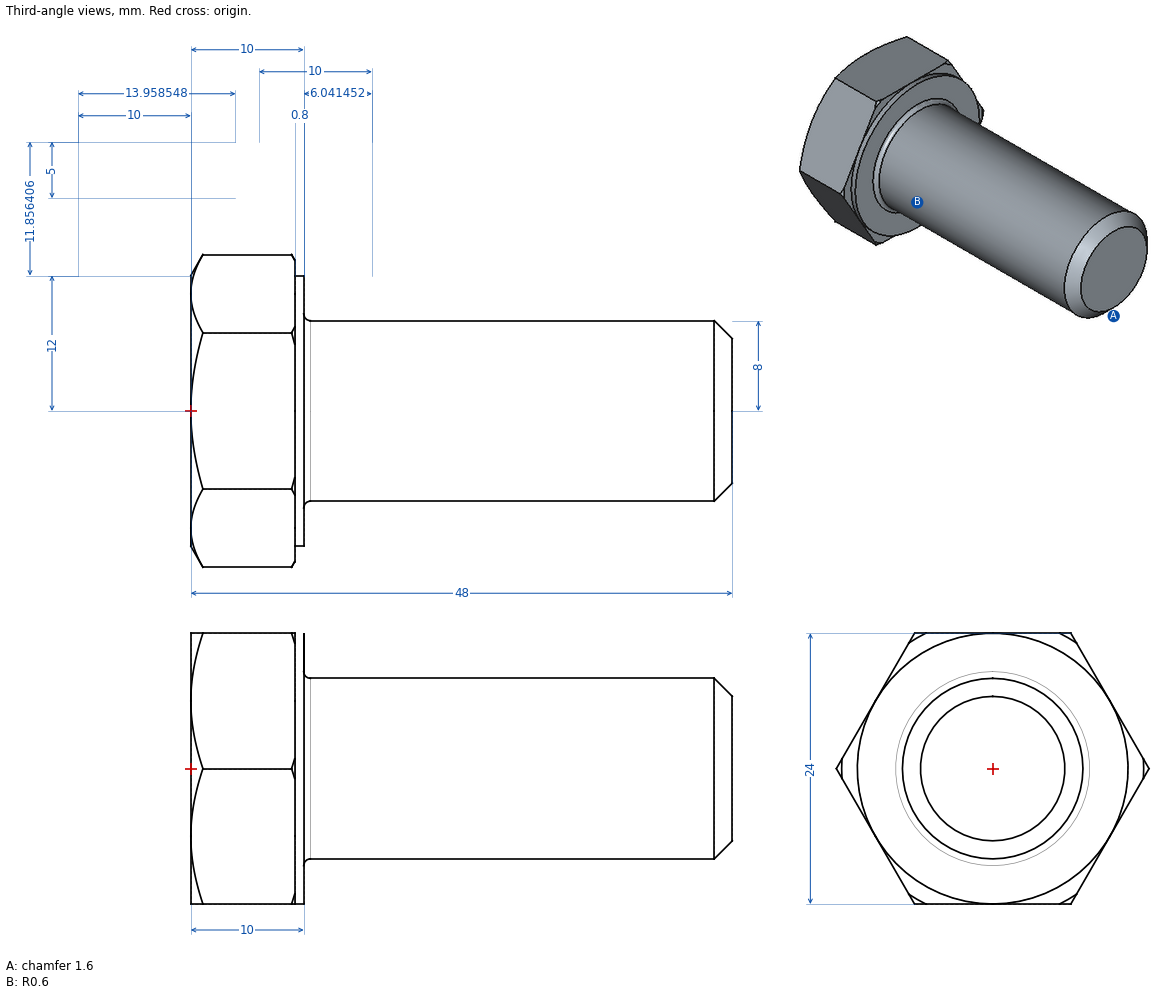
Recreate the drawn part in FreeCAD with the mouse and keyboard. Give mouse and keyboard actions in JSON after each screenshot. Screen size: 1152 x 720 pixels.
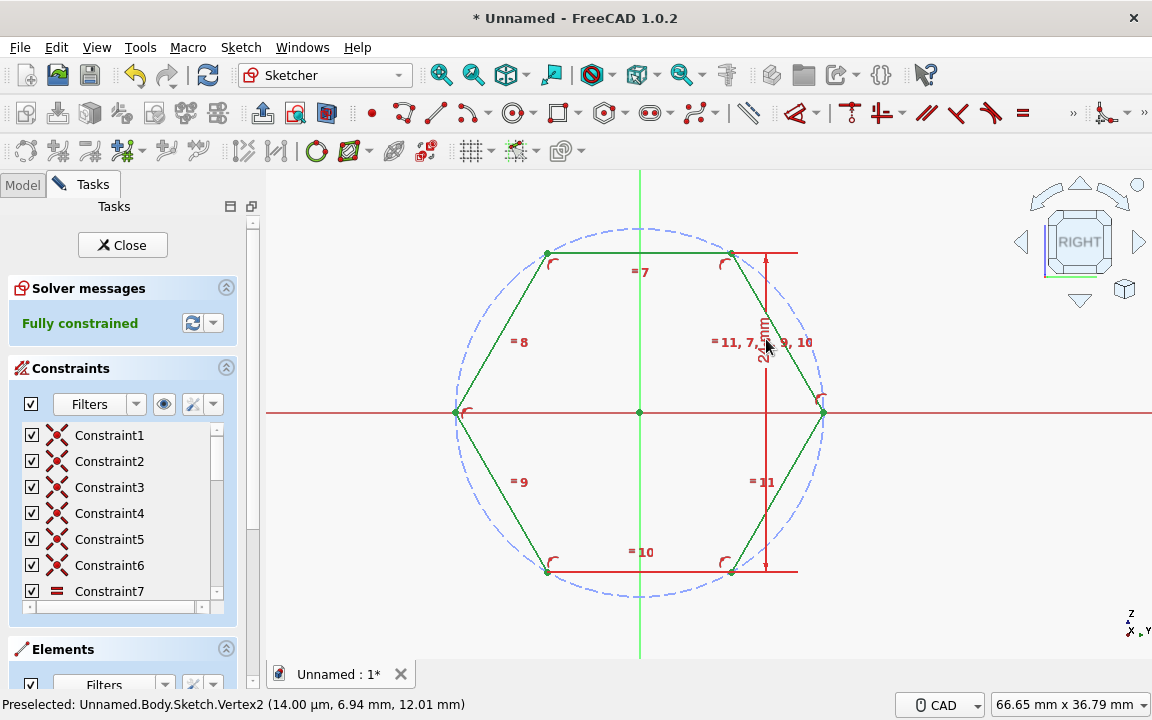
{"action": "left_click", "coordinate": [123, 245]}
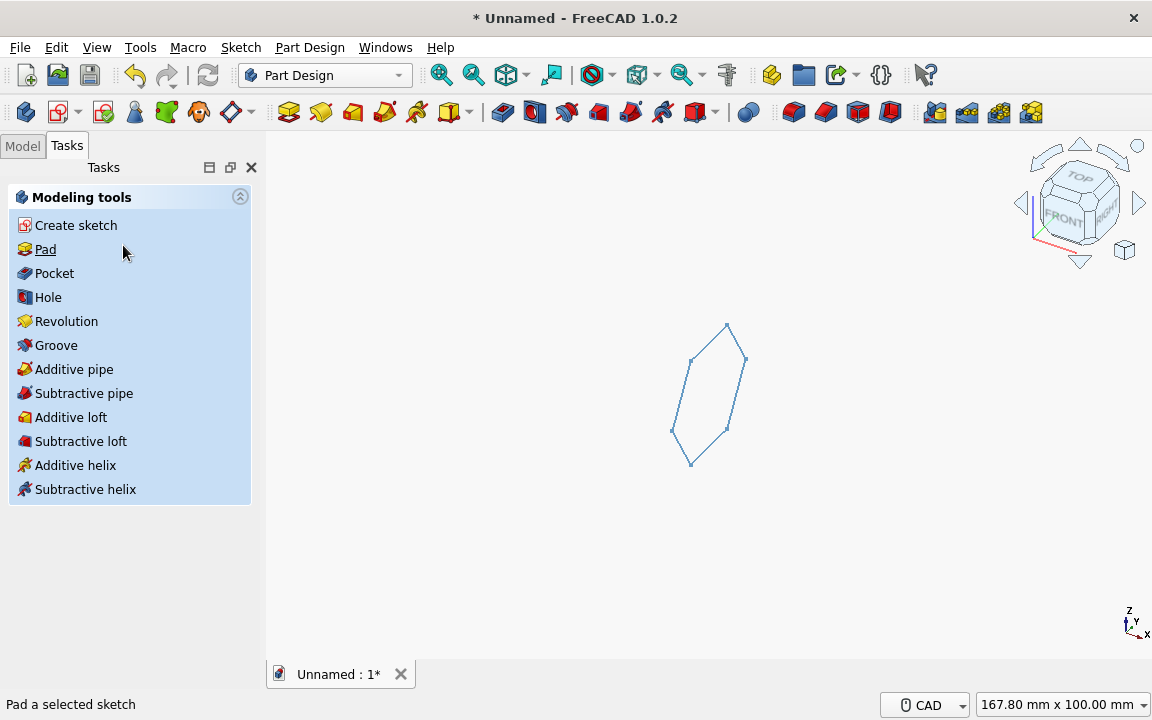
{"action": "left_click", "coordinate": [290, 112]}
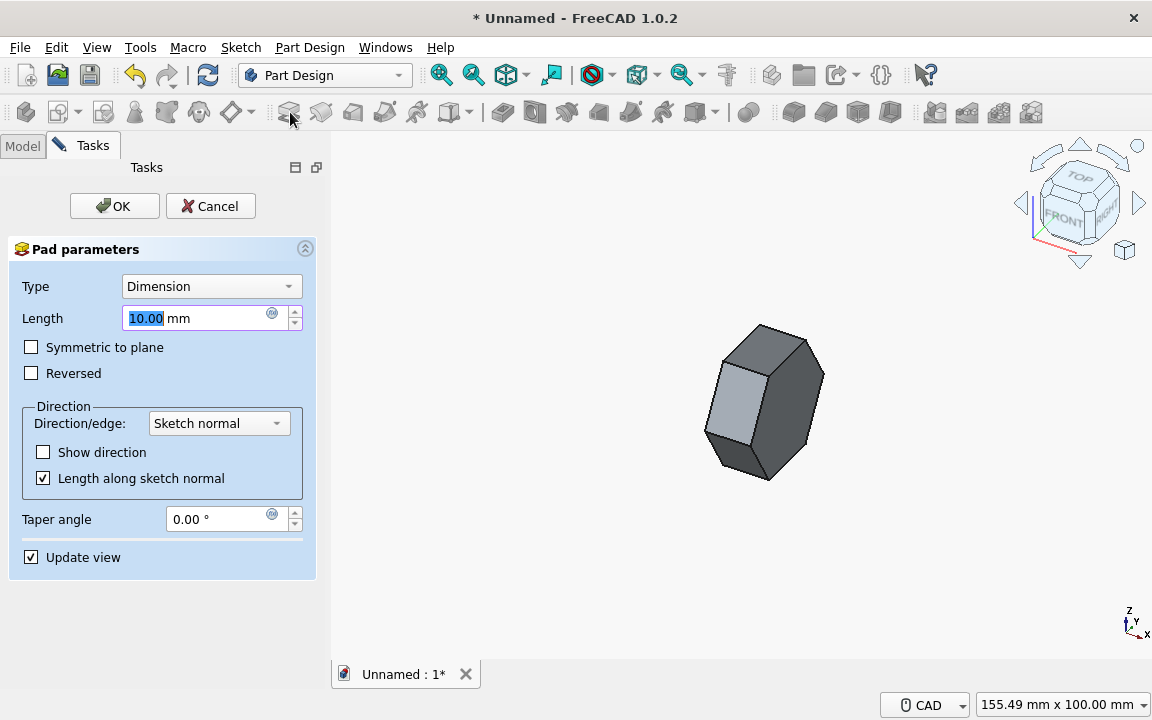
{"action": "type", "text": "10"}
{"action": "key", "text": "Tab"}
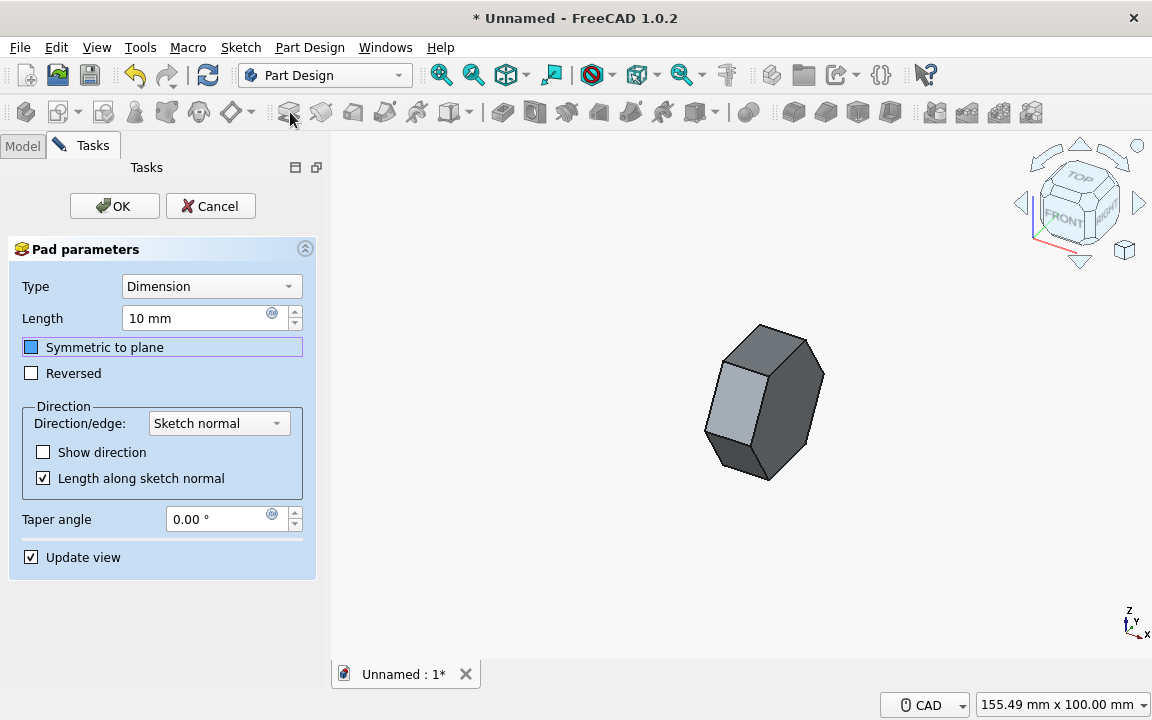
{"action": "left_click", "coordinate": [115, 206]}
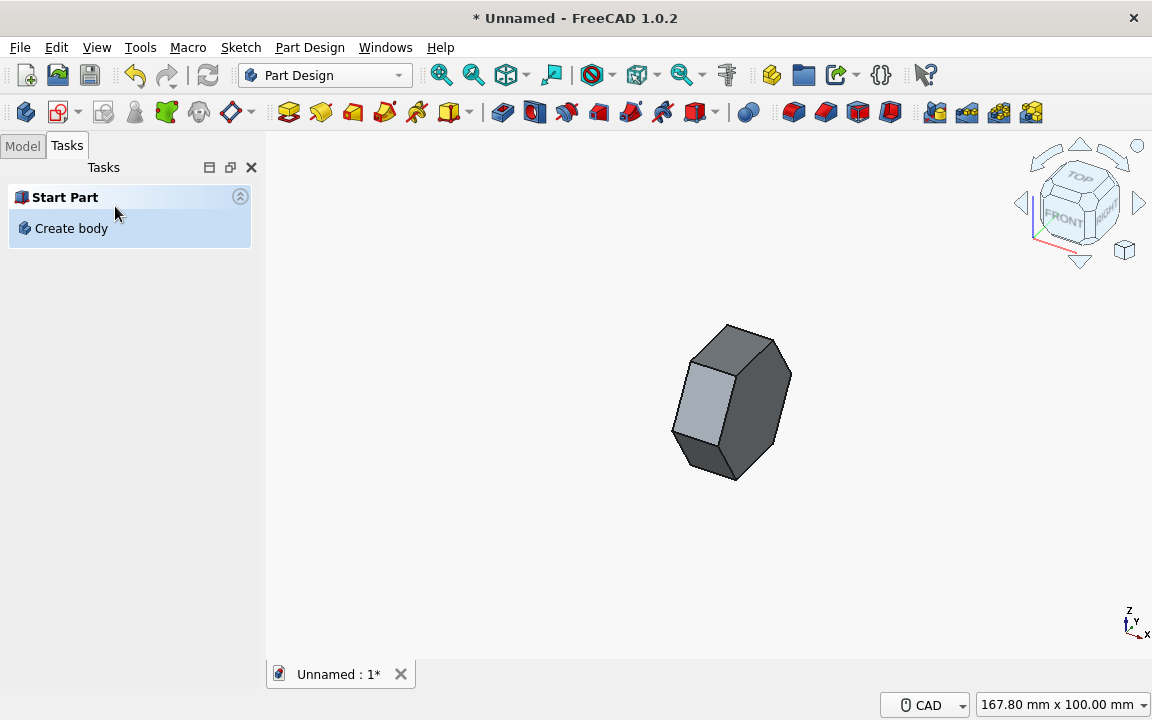
{"action": "left_click", "coordinate": [442, 76]}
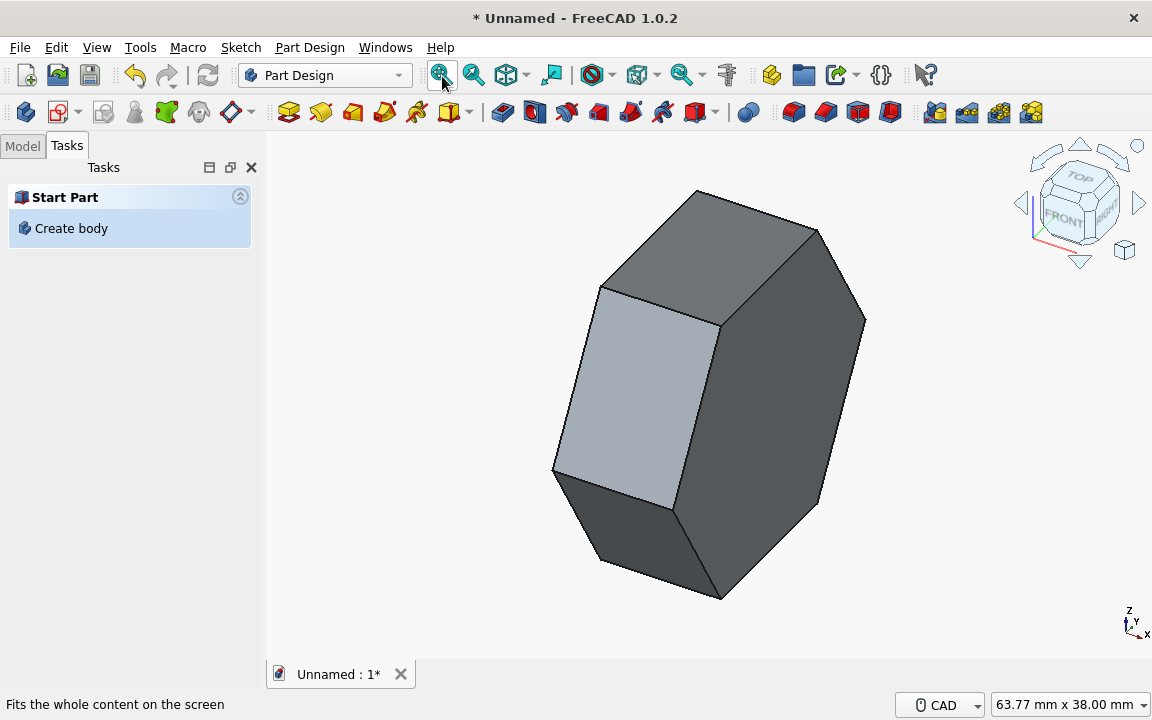
{"action": "left_click", "coordinate": [58, 112]}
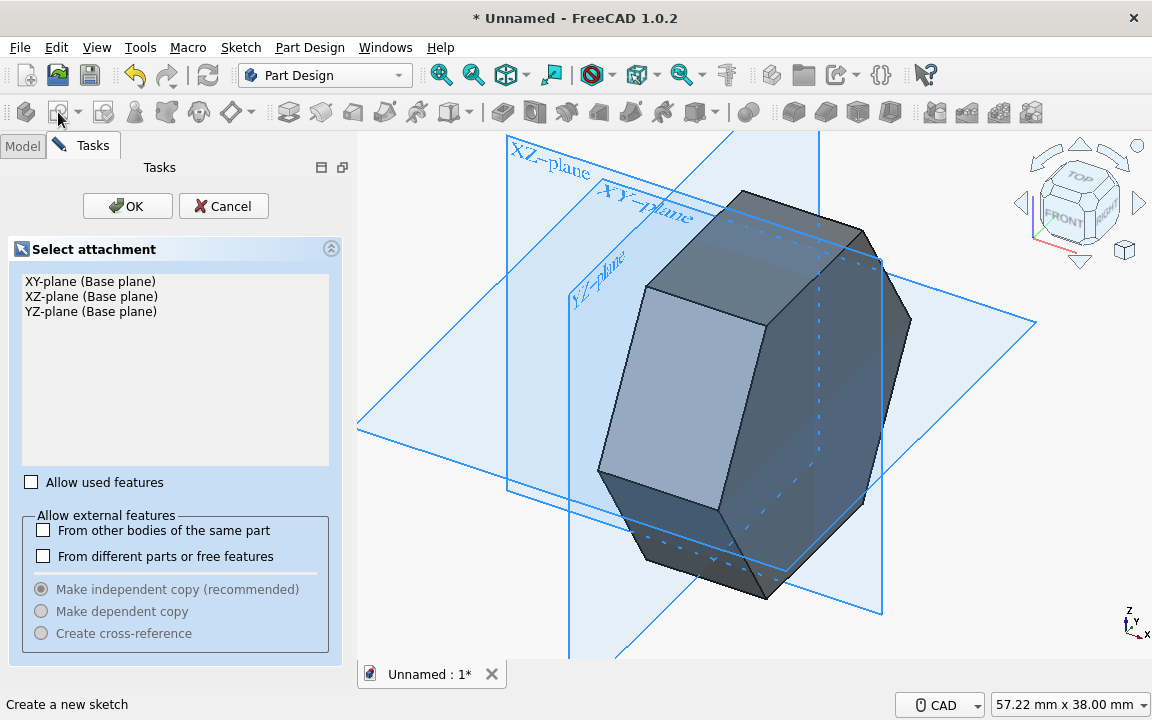
{"action": "left_click", "coordinate": [82, 282]}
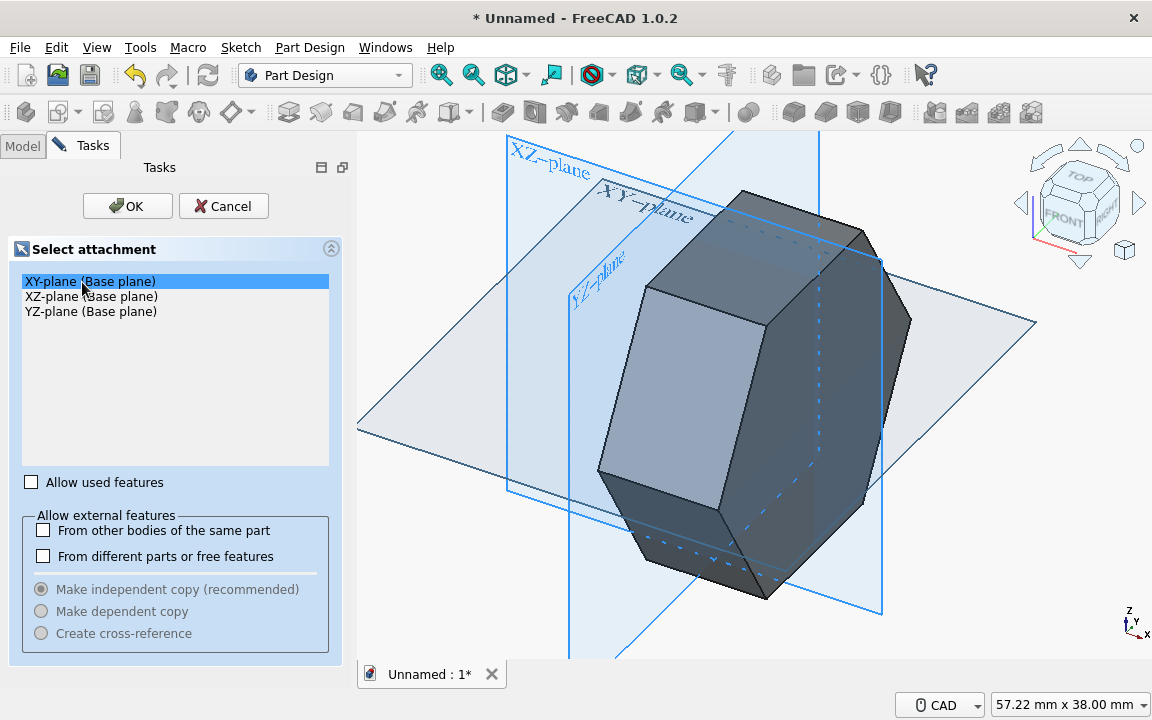
{"action": "left_click", "coordinate": [128, 206]}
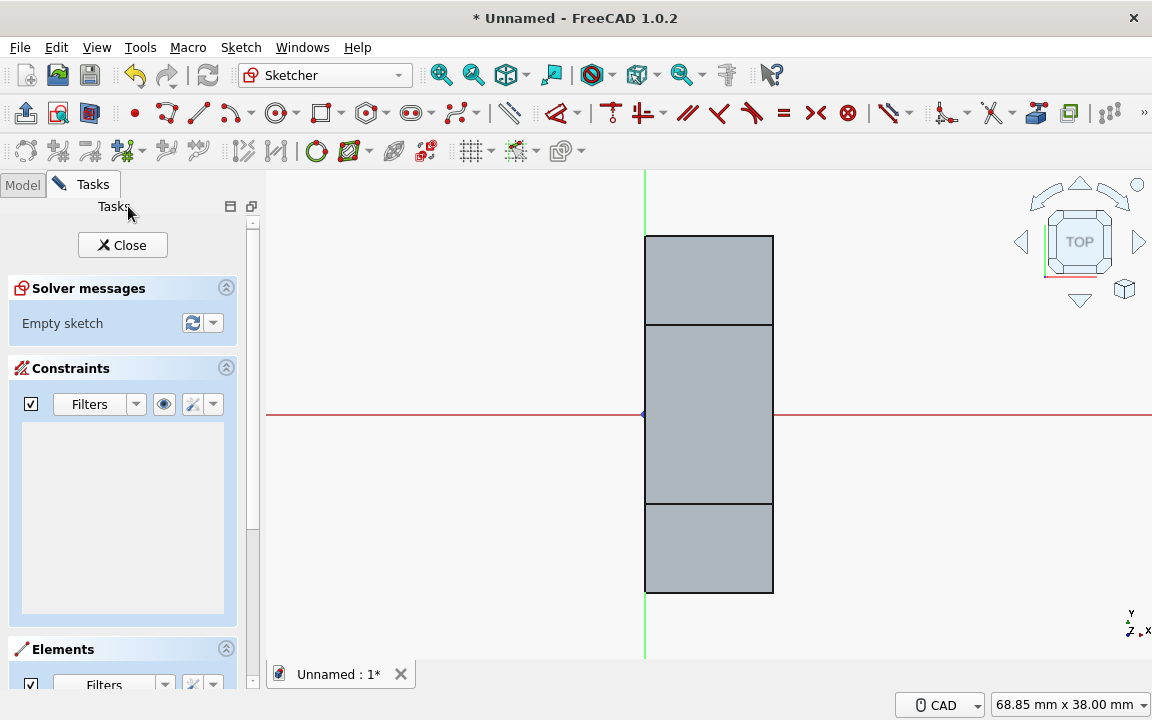
{"action": "left_click", "coordinate": [90, 114]}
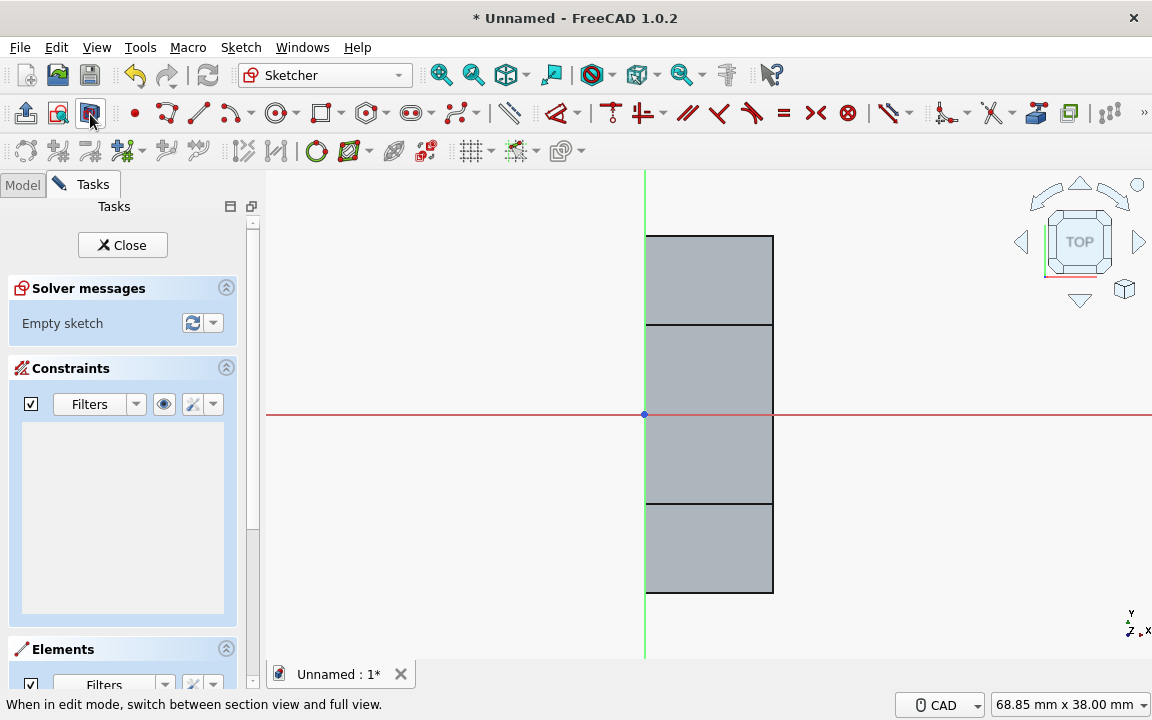
{"action": "scroll", "coordinate": [294, 519], "scroll_direction": "down", "scroll_amount": 2}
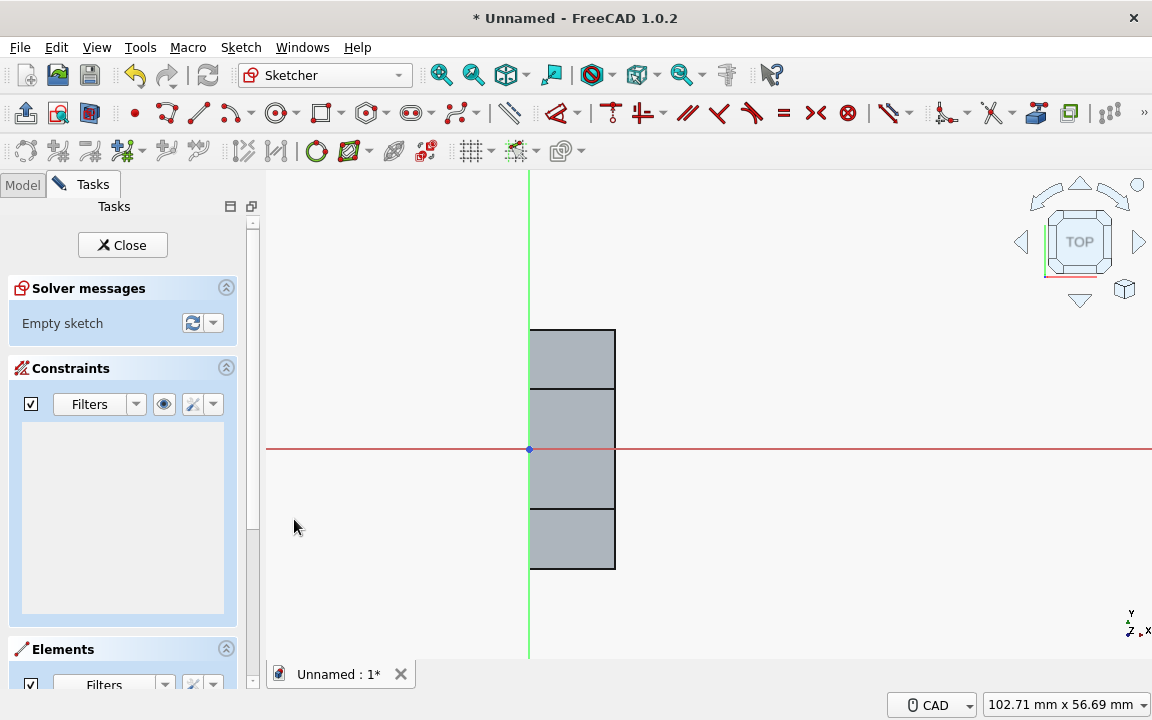
{"action": "left_click", "coordinate": [322, 114]}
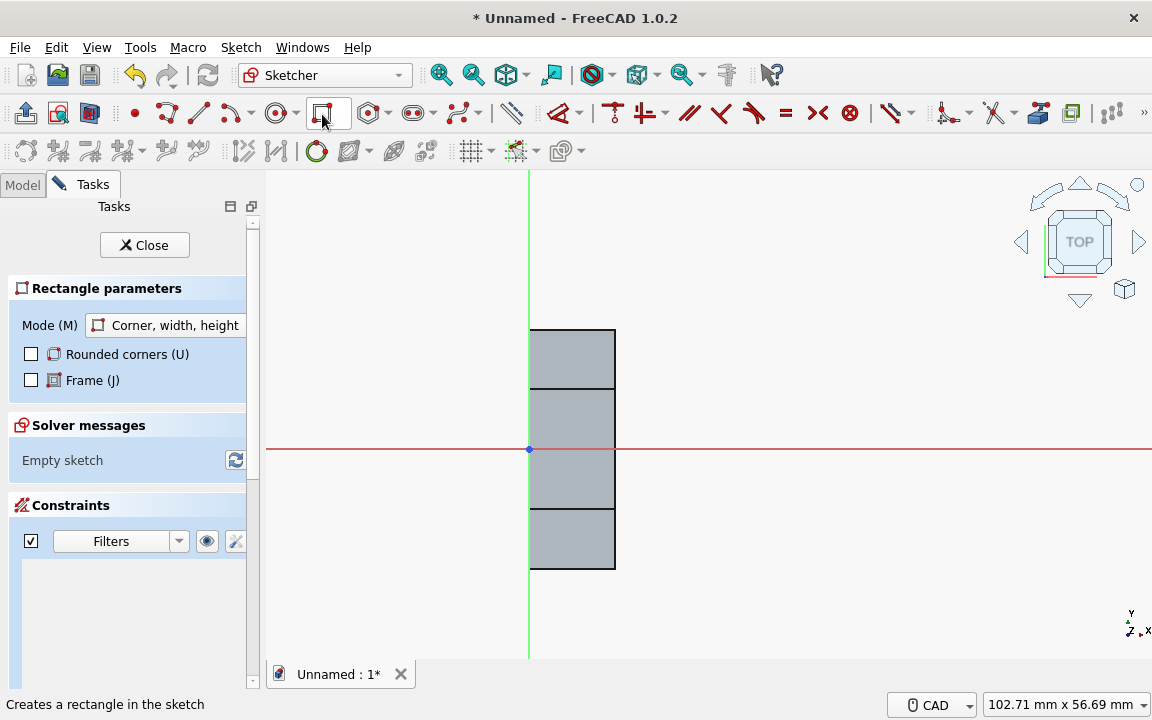
{"action": "left_click", "coordinate": [529, 449]}
{"action": "mouse_move", "coordinate": [943, 380]}